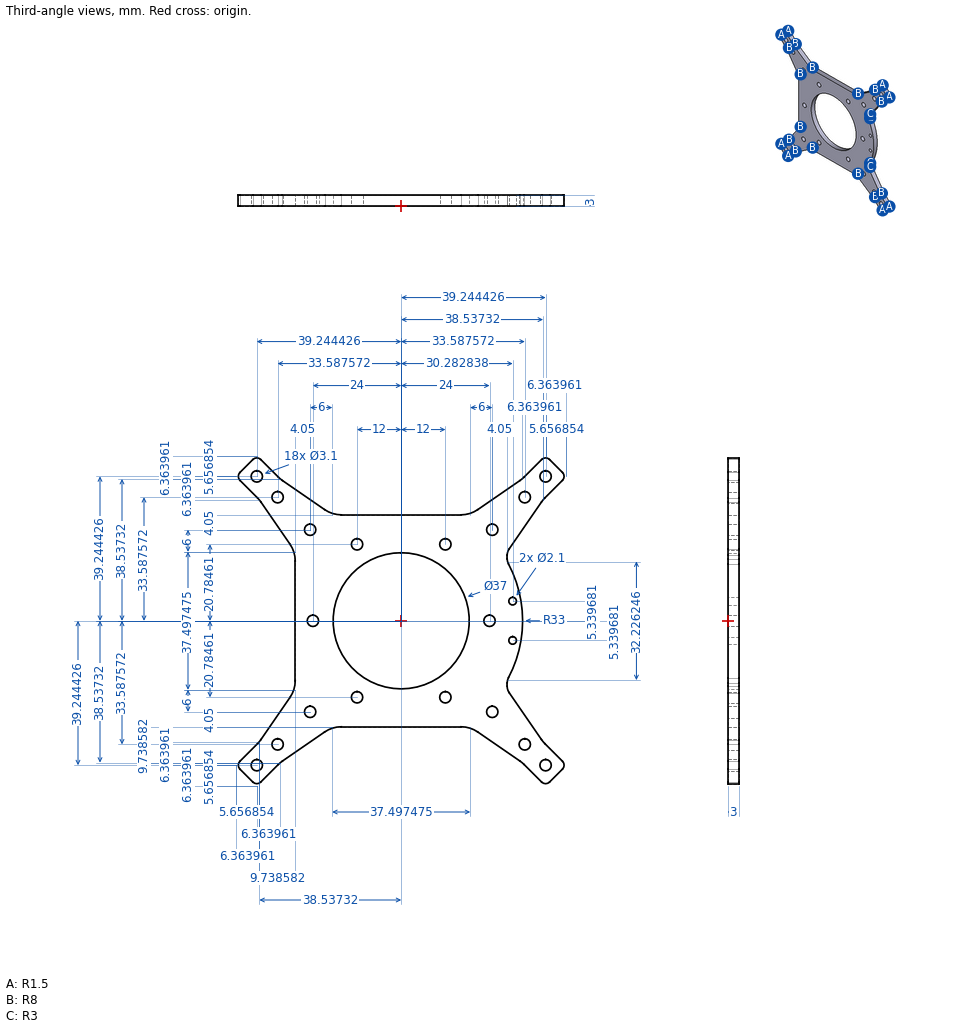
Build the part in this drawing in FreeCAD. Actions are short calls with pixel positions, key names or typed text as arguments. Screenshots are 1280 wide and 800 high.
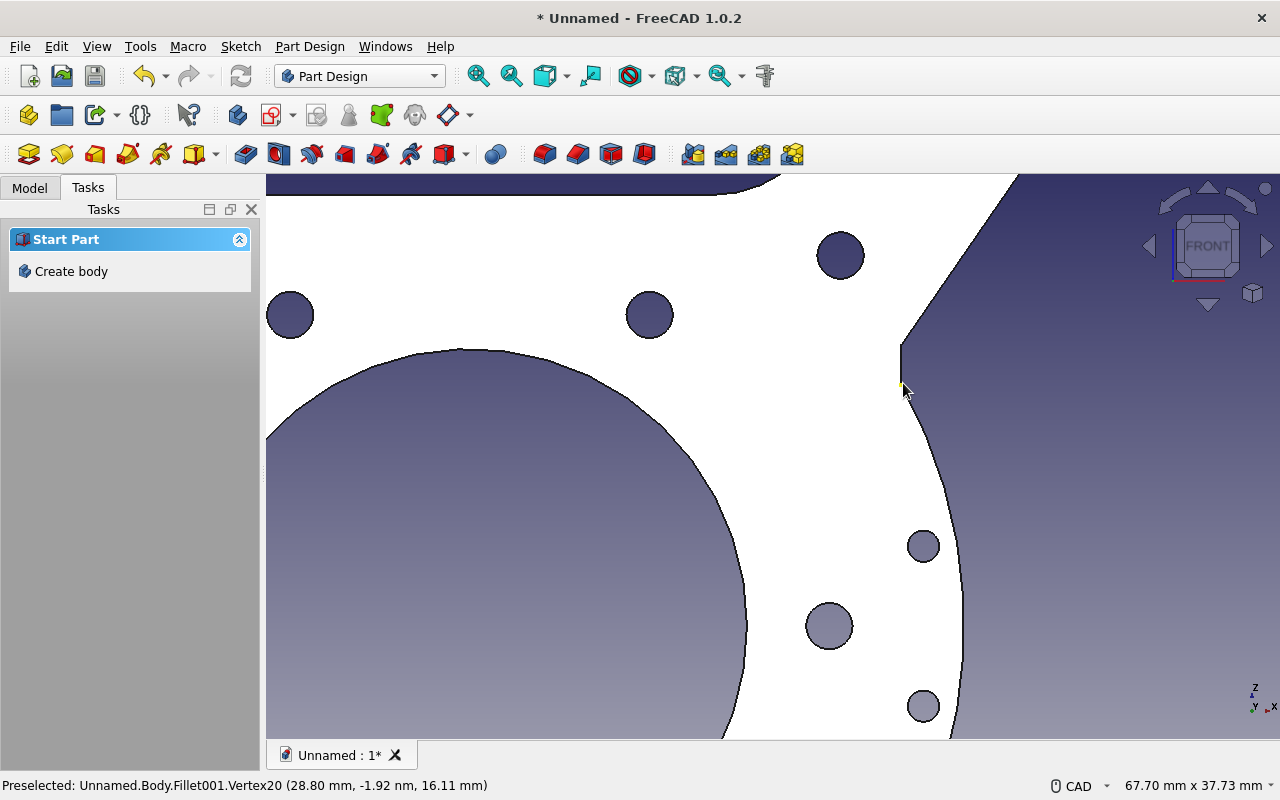
click(479, 76)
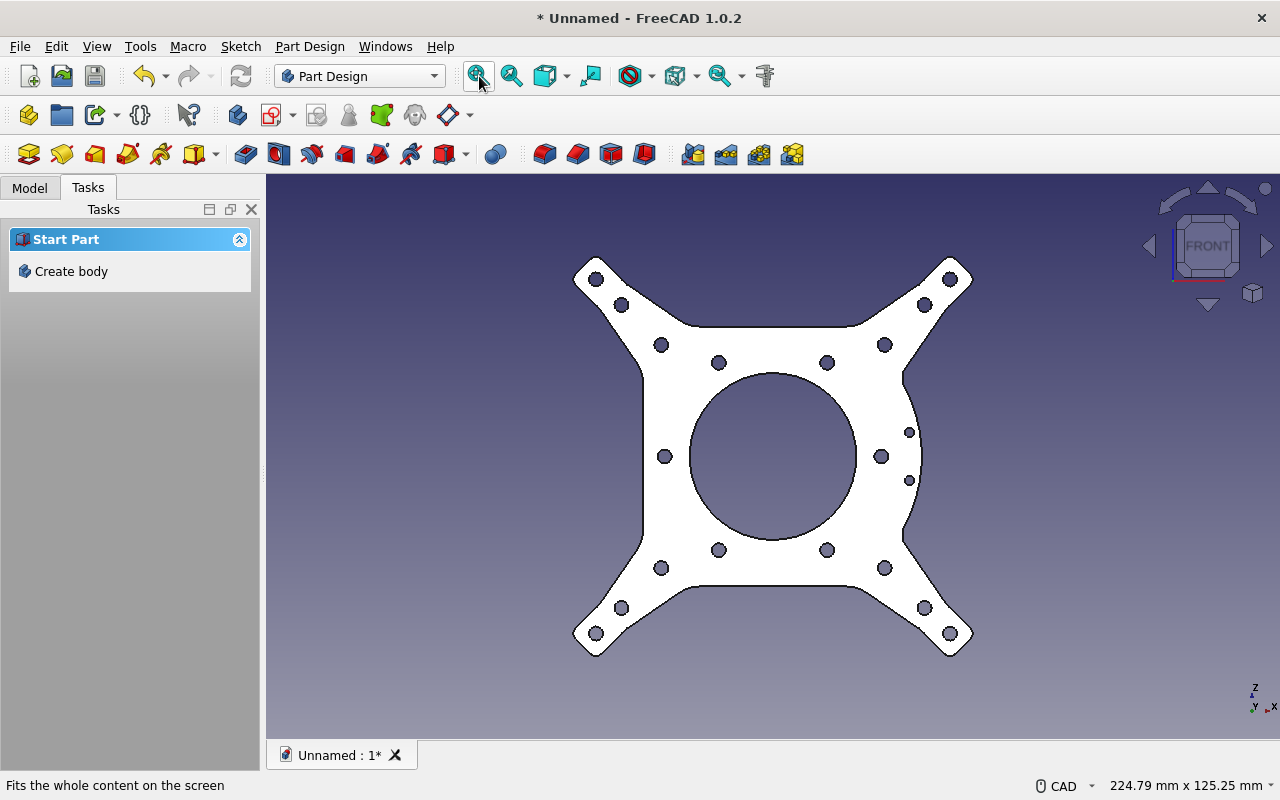
key(3)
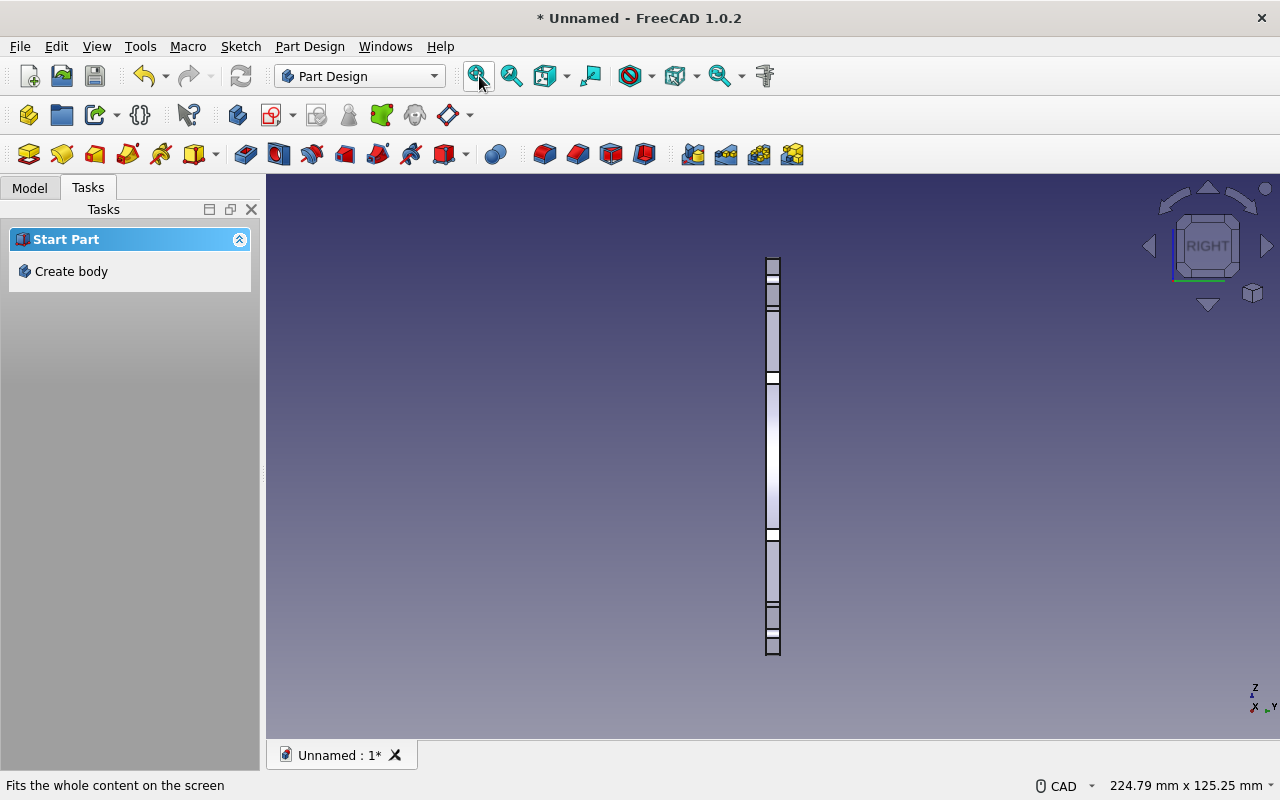
scroll(773, 383, up, 6)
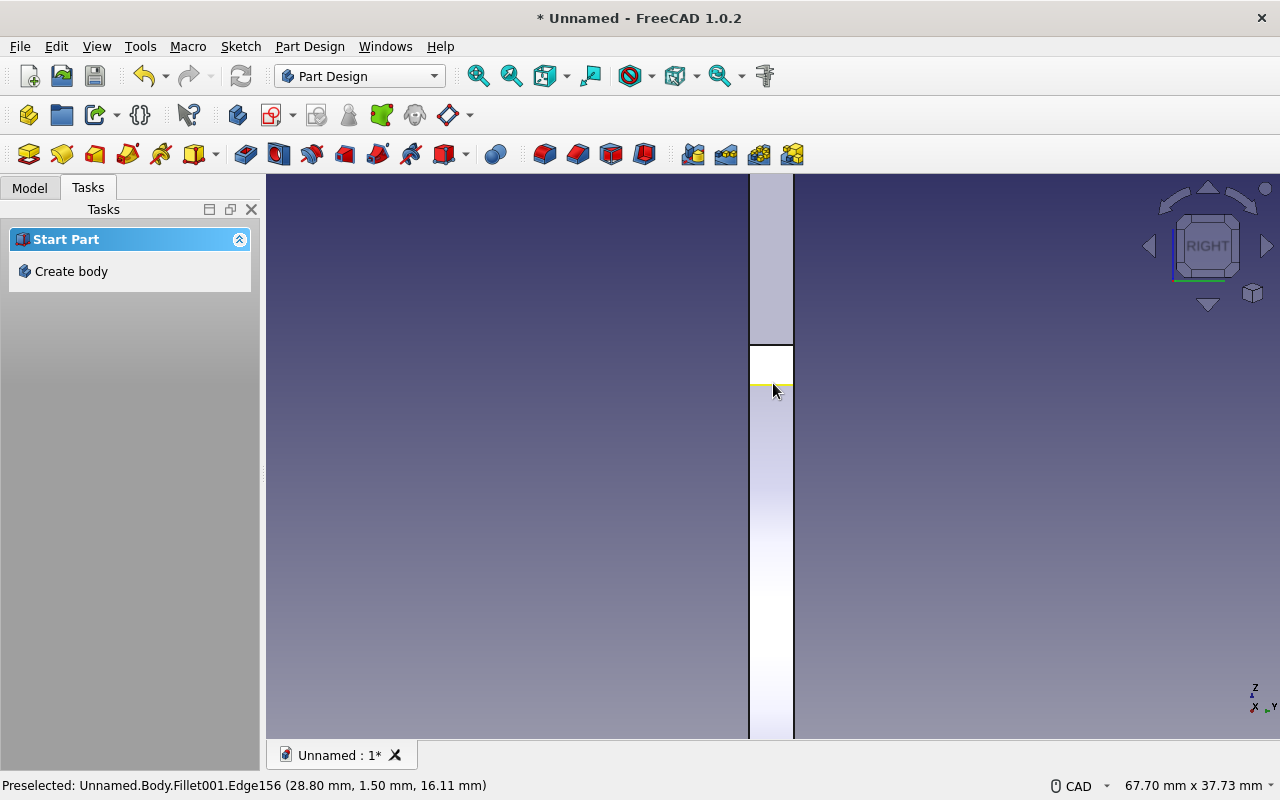
key(v)
key(f)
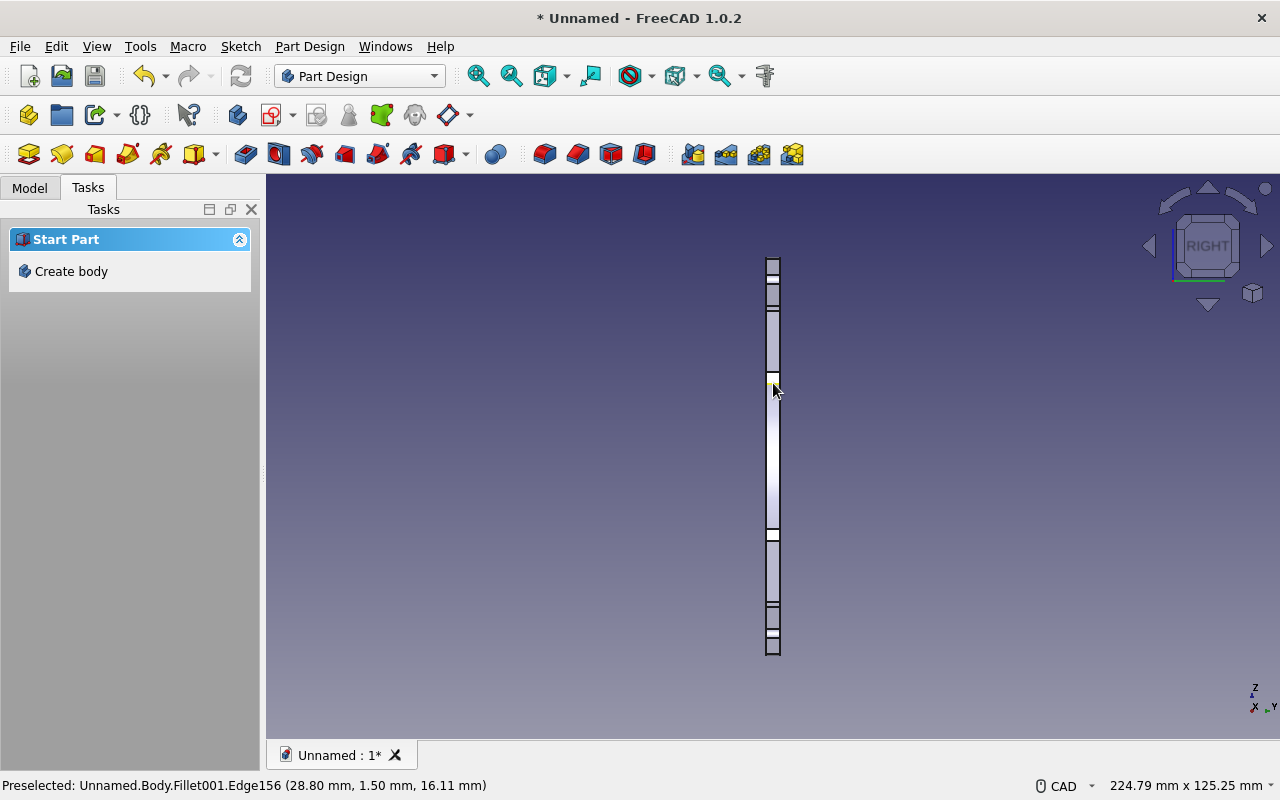
key(5)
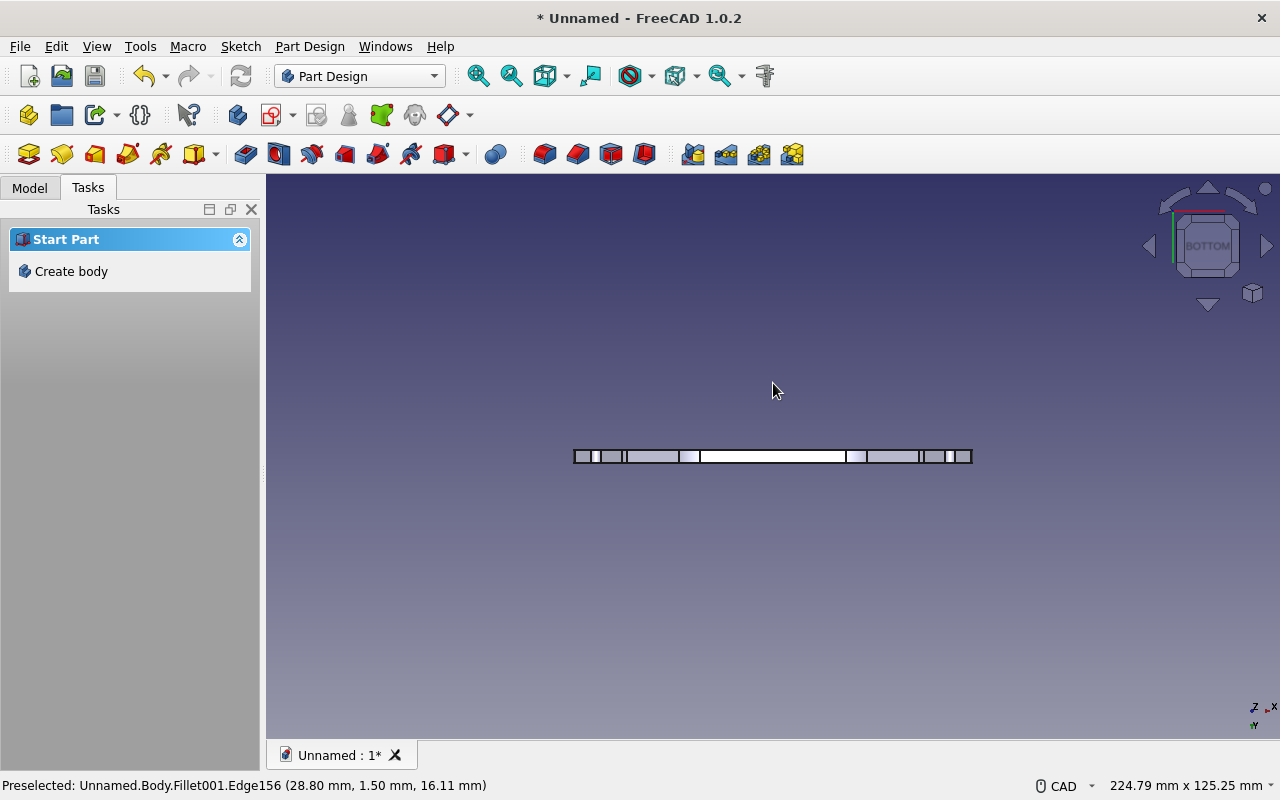
click(479, 76)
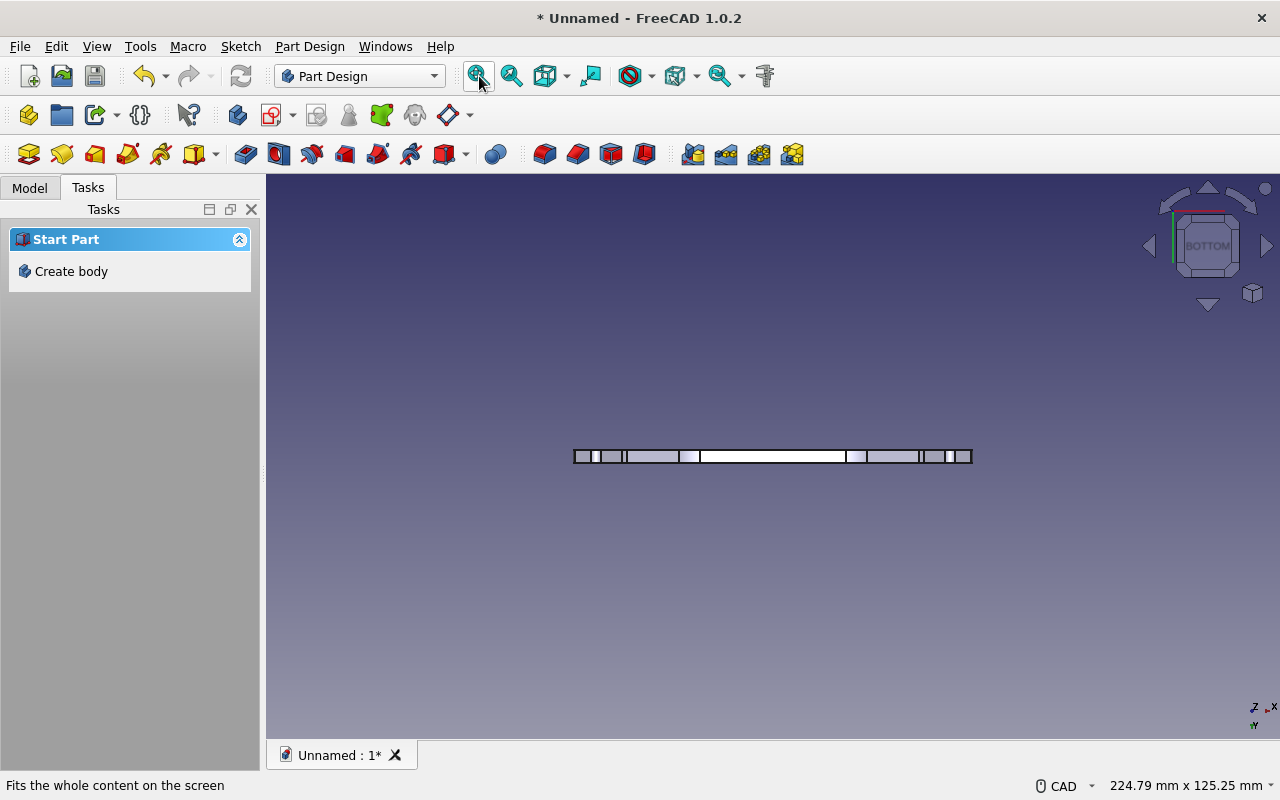
scroll(903, 455, up, 6)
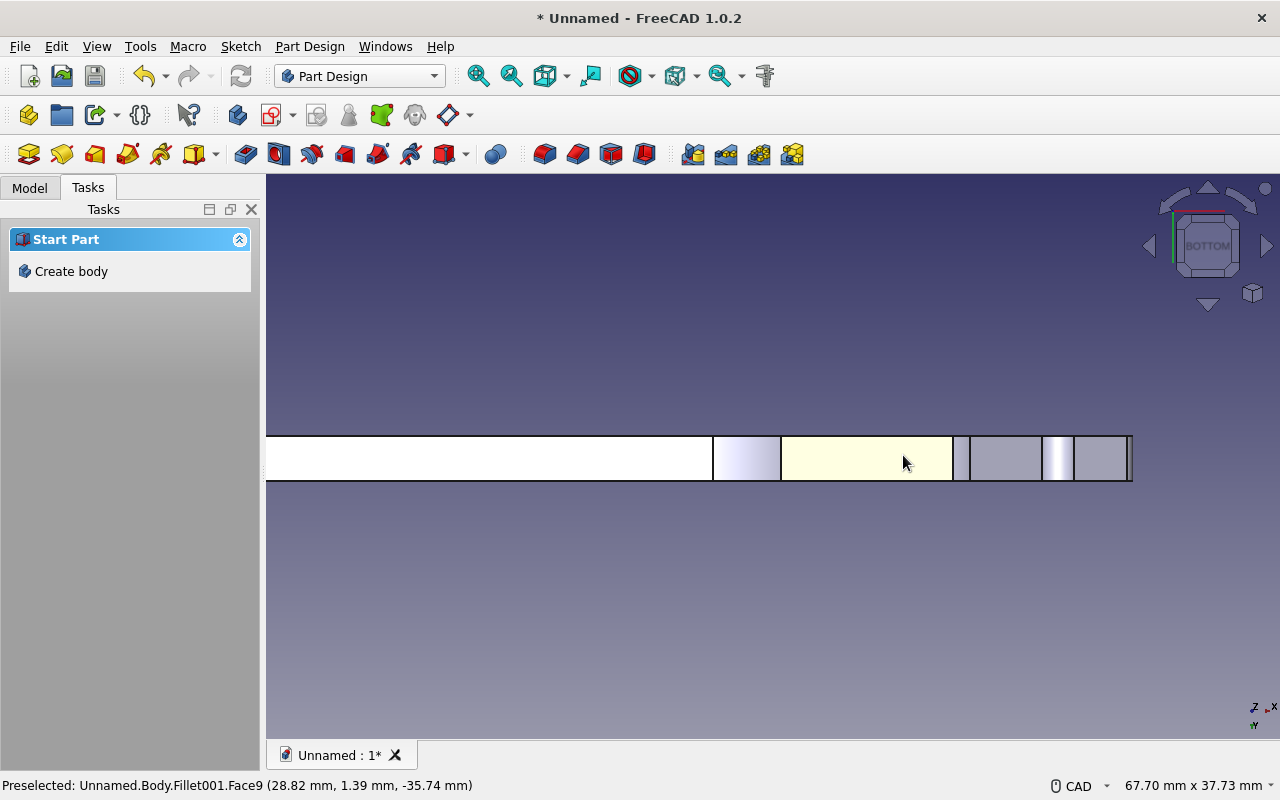
key(v)
key(f)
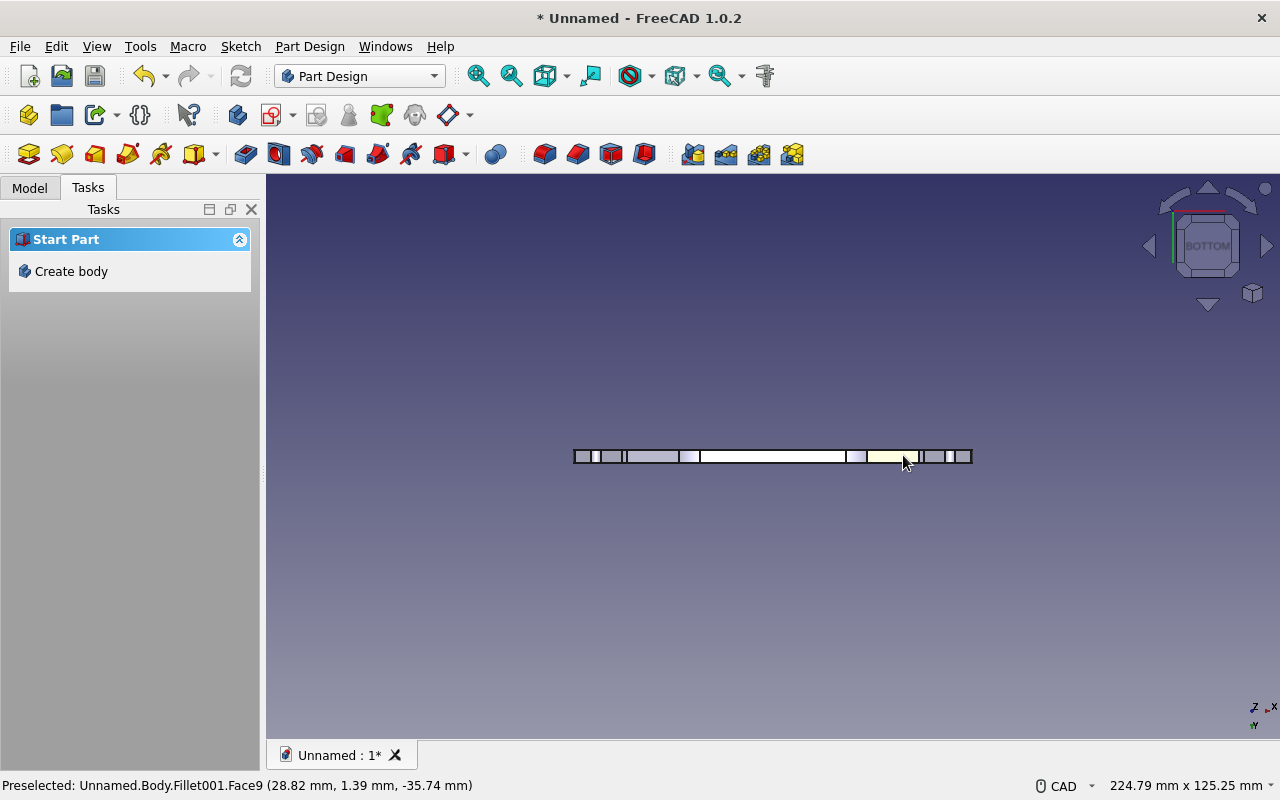
key(4)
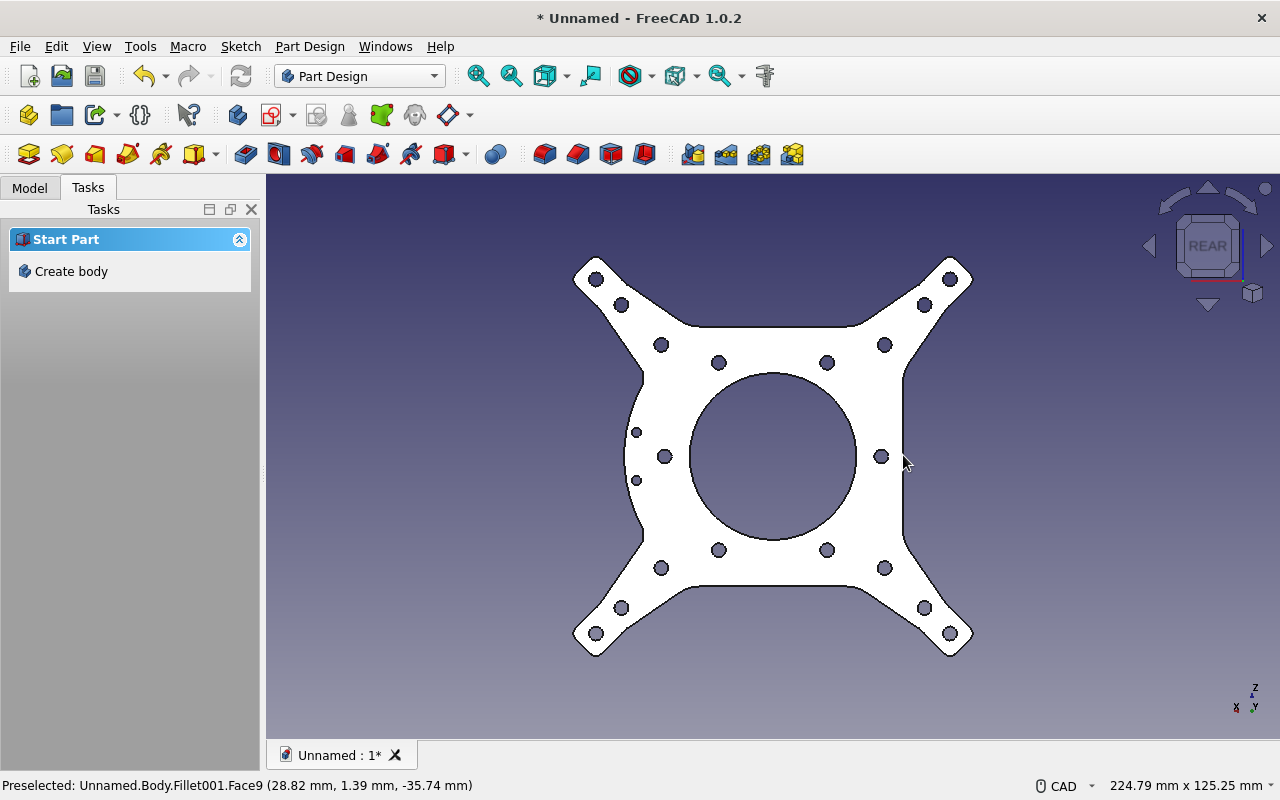
scroll(643, 383, up, 6)